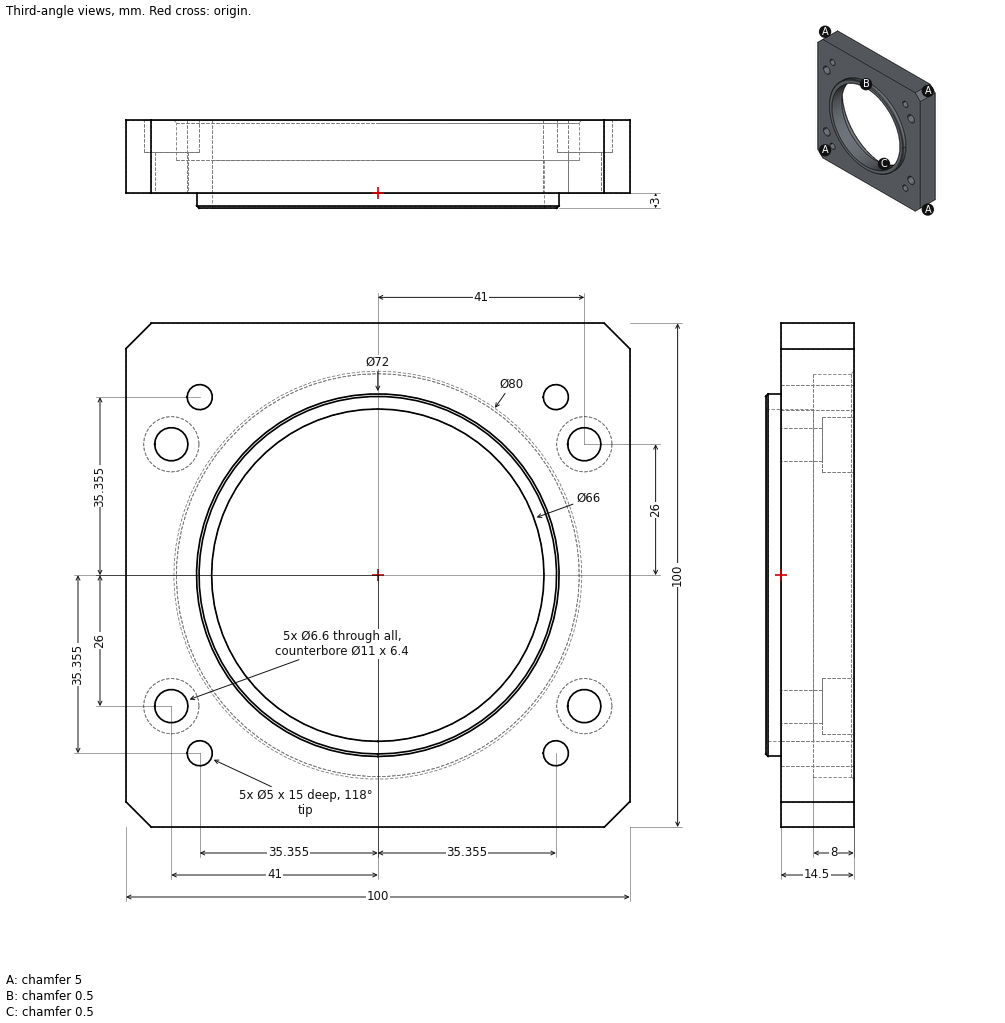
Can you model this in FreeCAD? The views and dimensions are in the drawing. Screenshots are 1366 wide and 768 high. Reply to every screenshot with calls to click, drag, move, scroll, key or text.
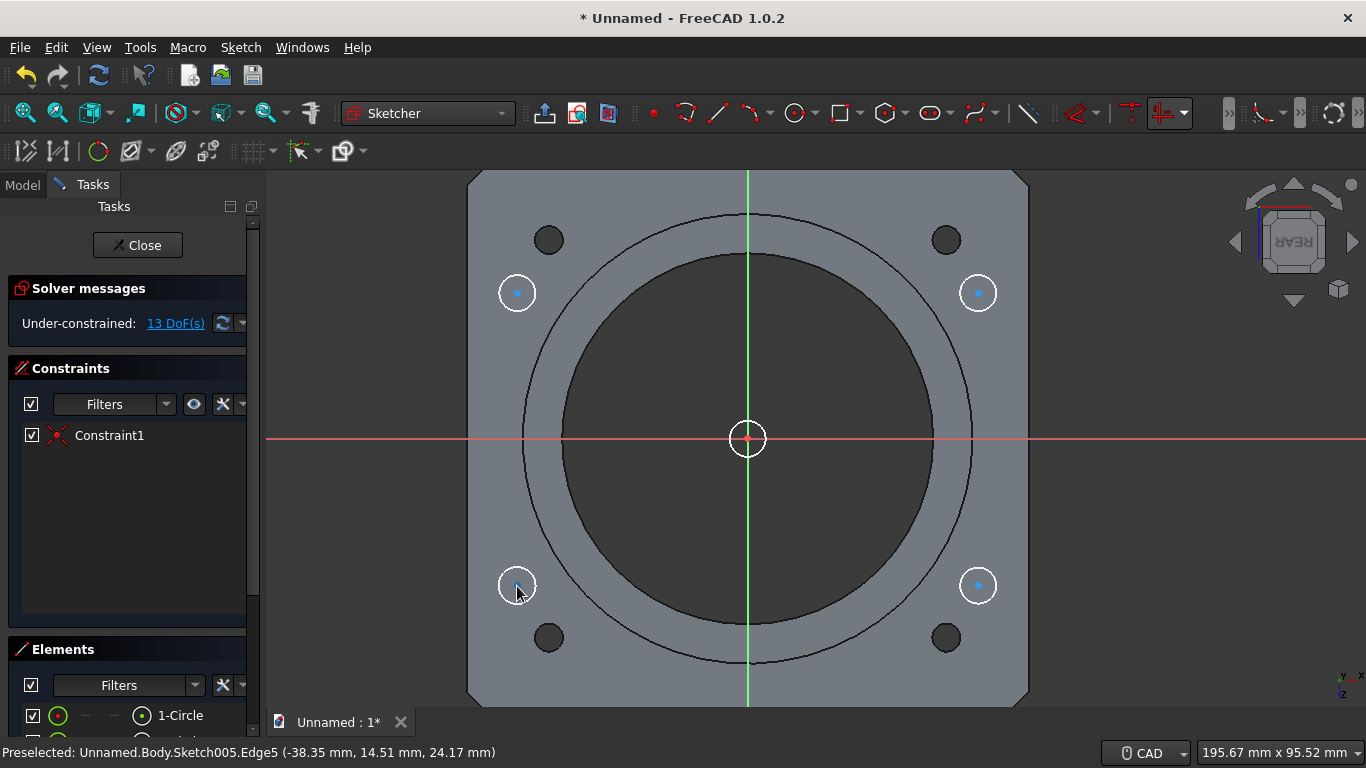
click(530, 280)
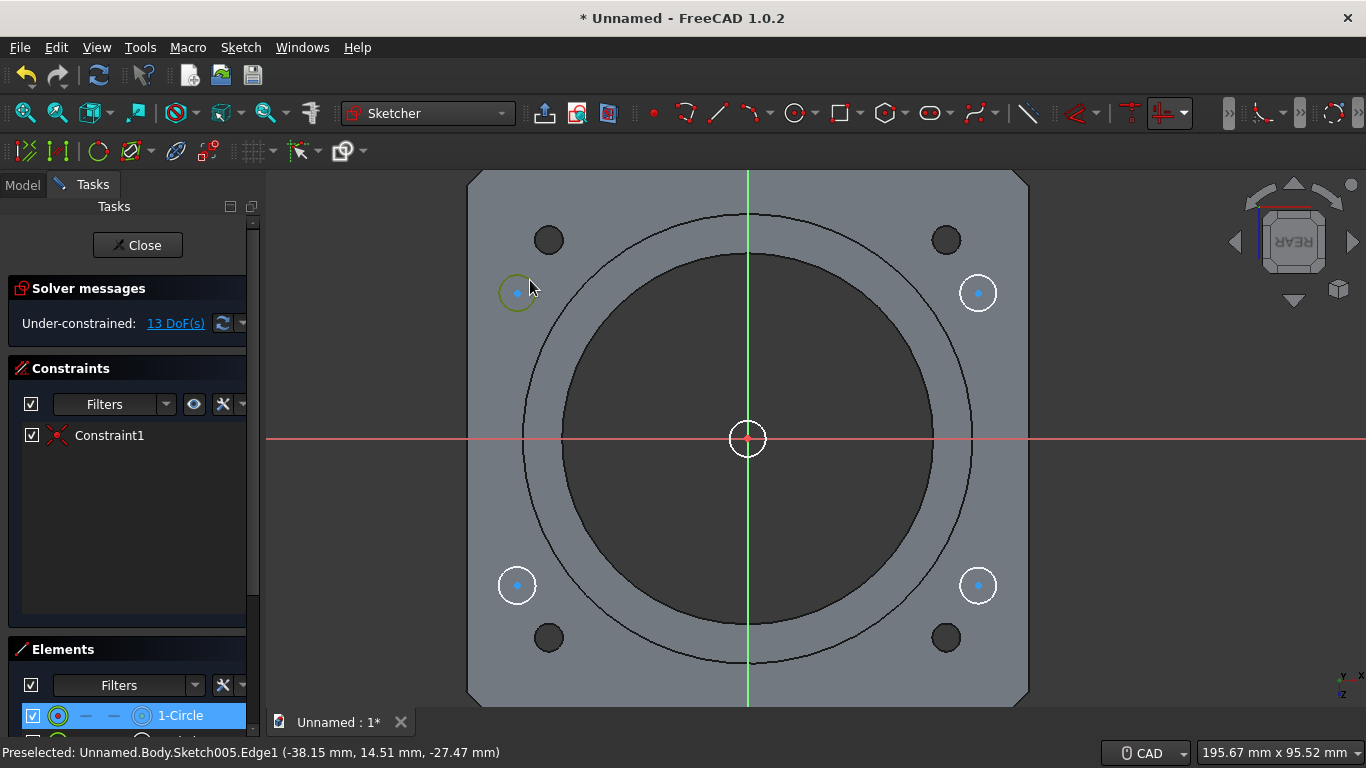
click(760, 426)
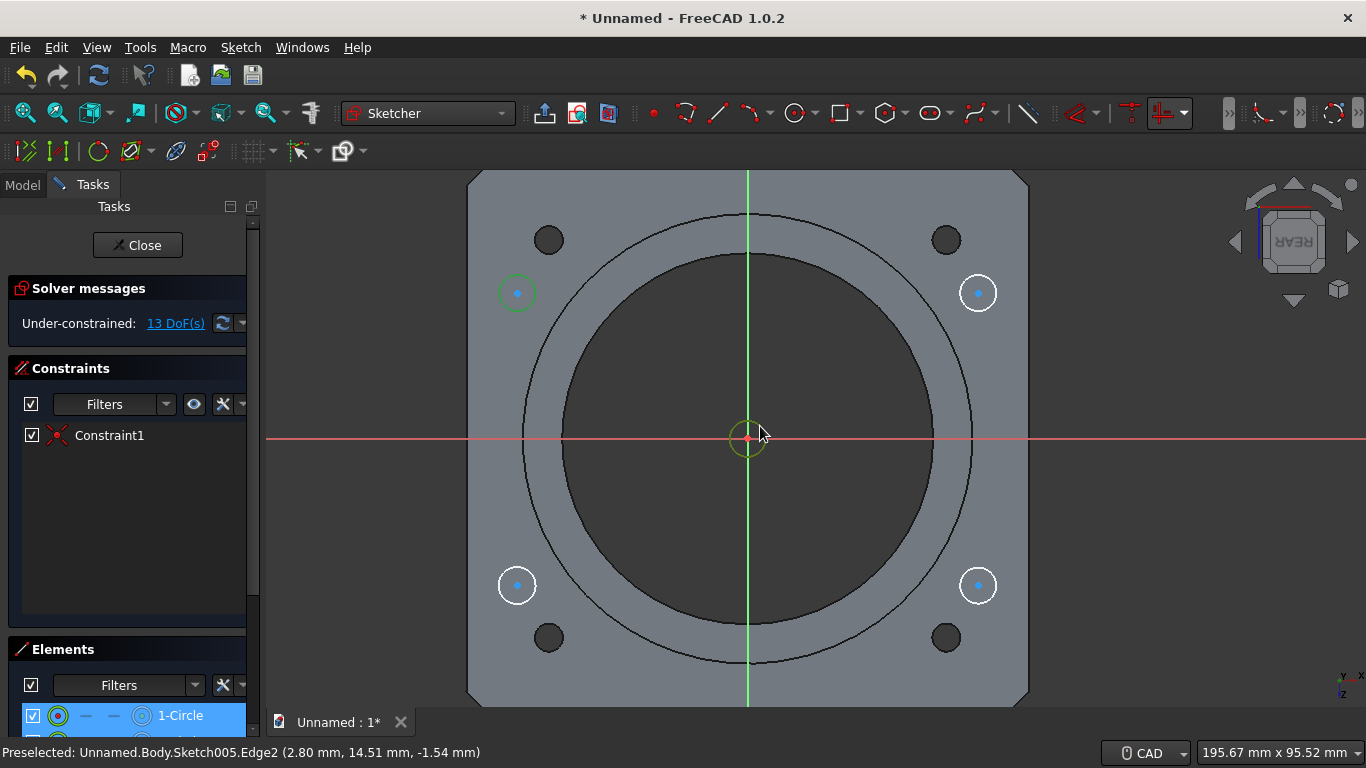
click(991, 573)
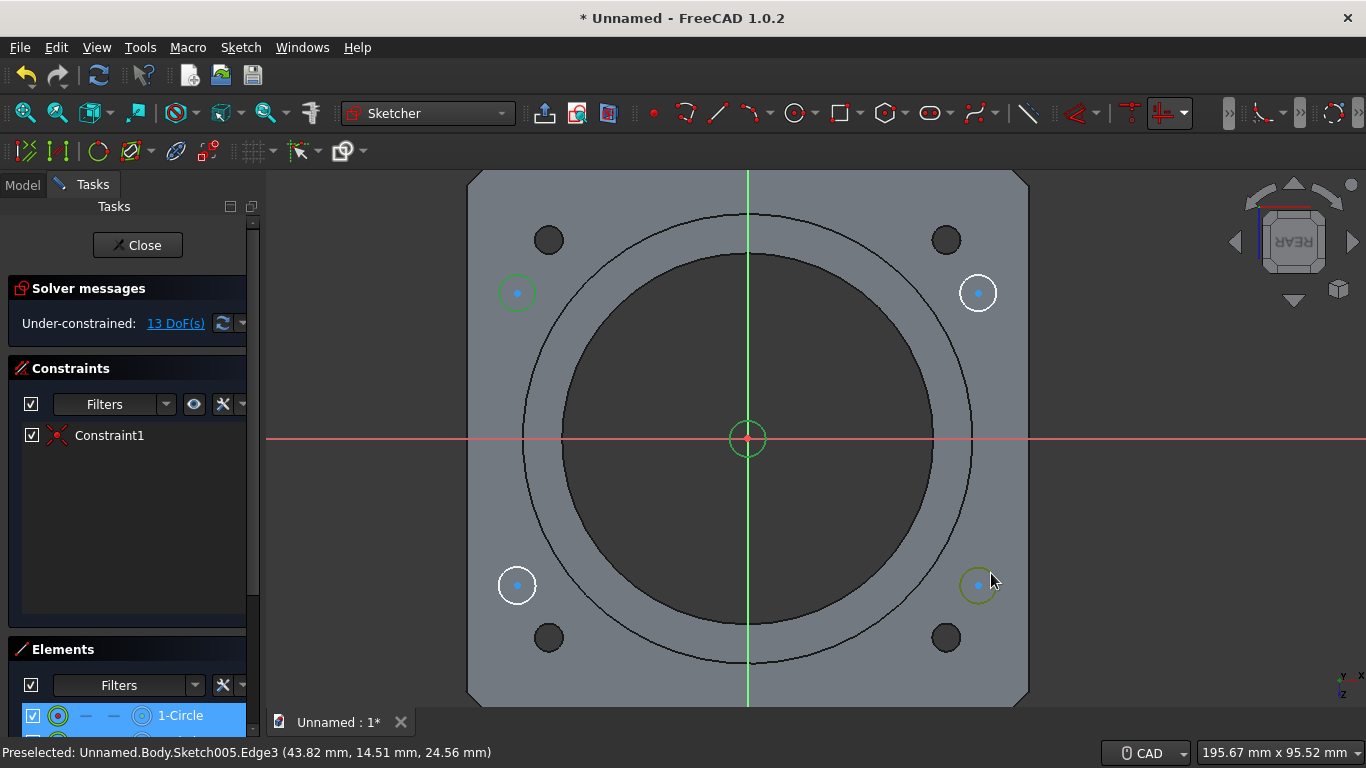
click(991, 280)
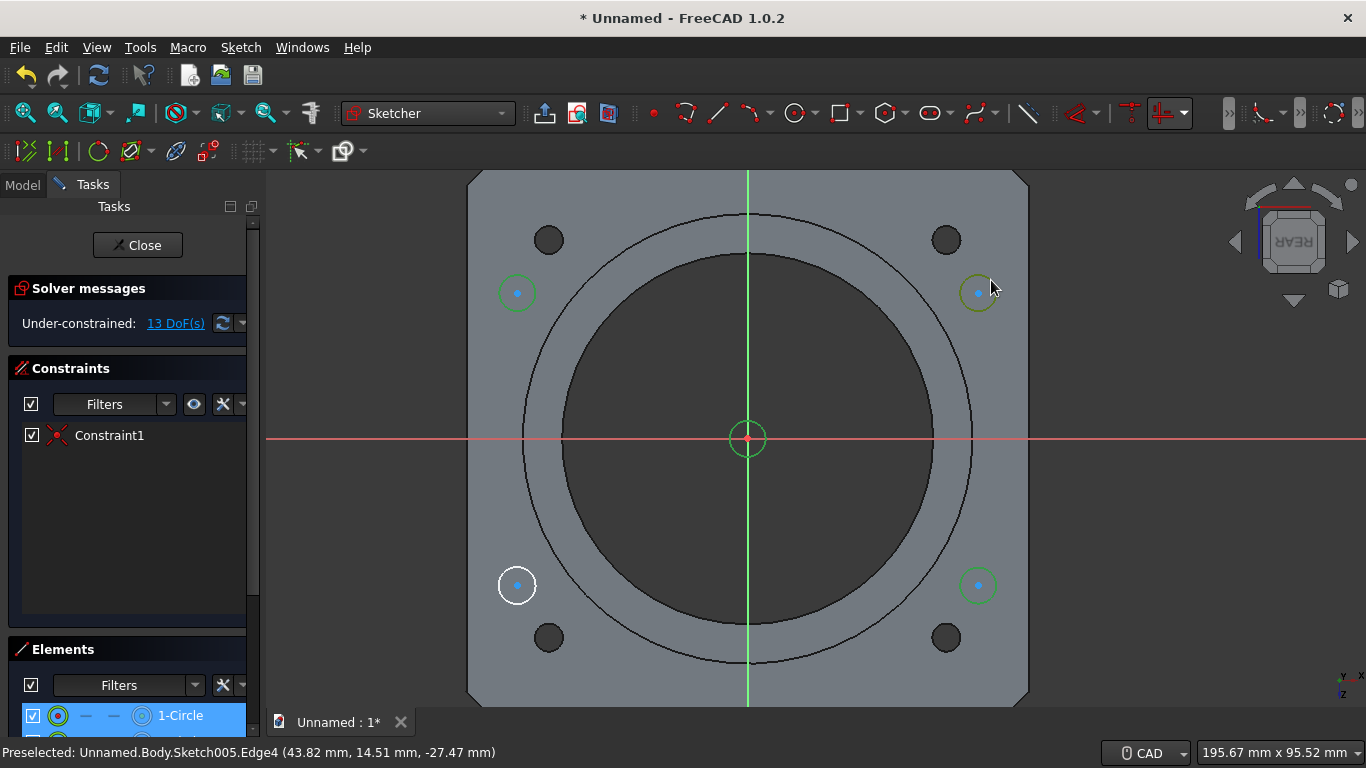
click(530, 572)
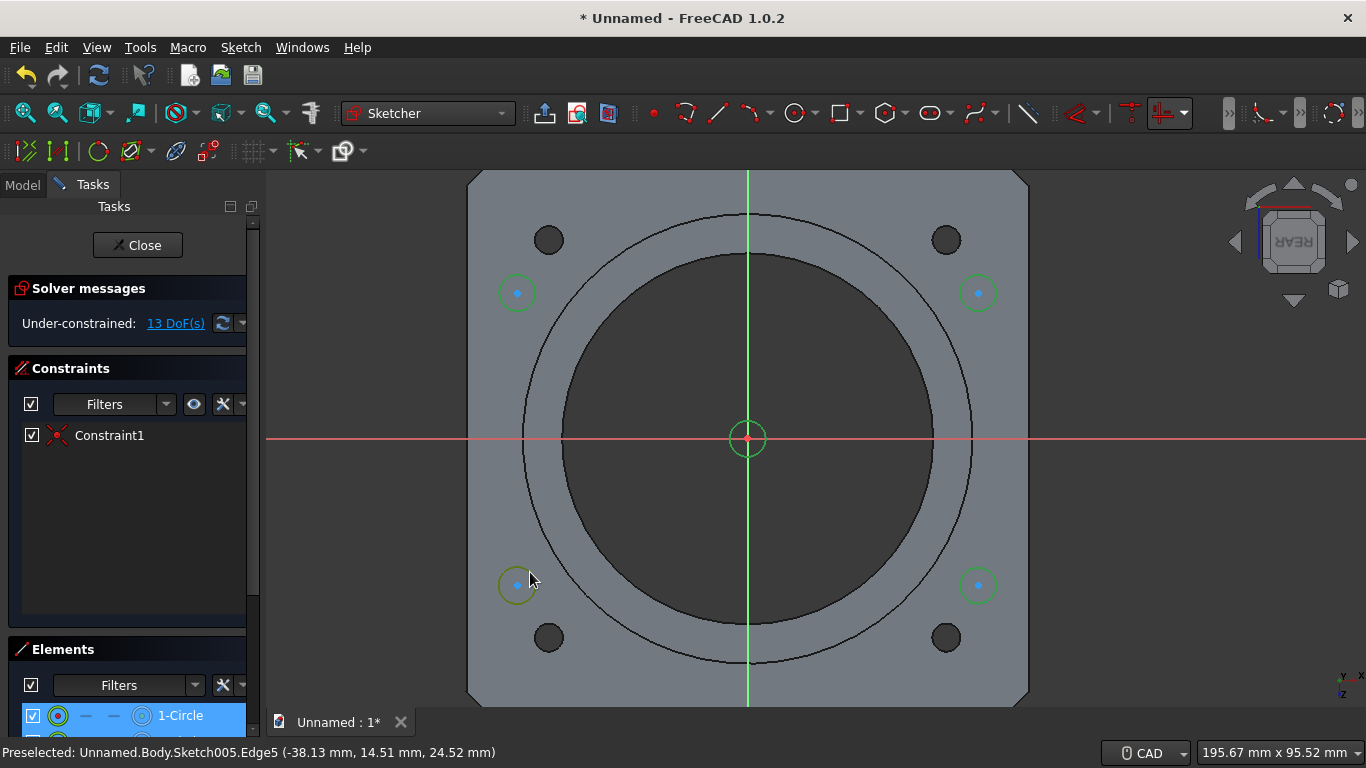
key(e)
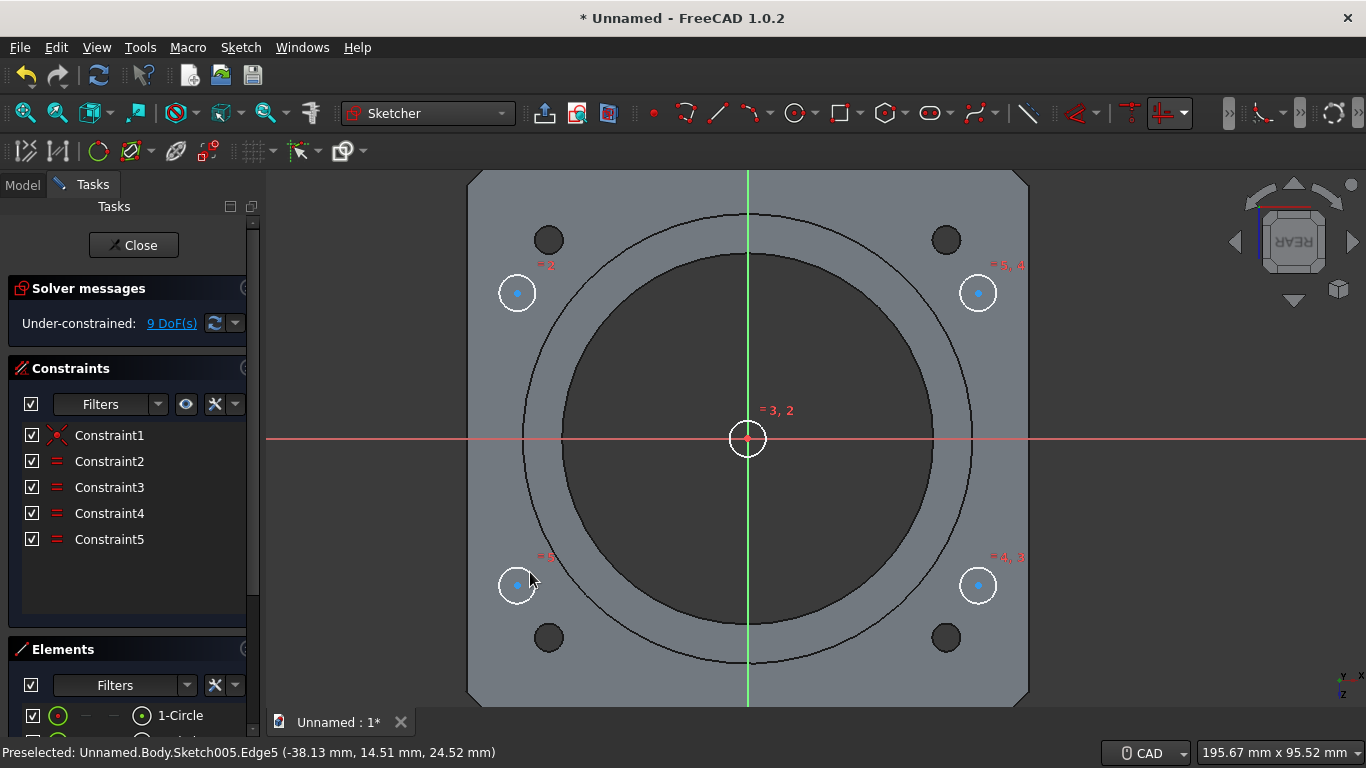
click(978, 586)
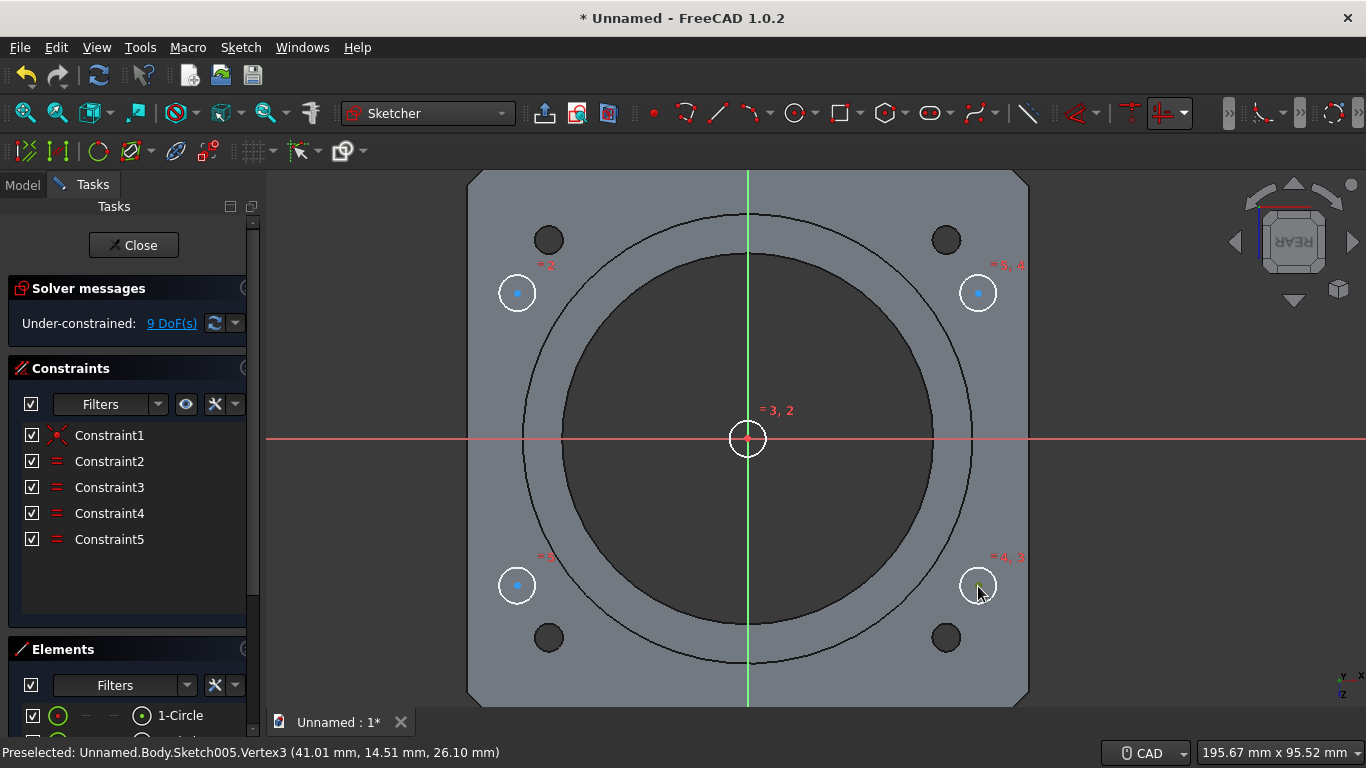
click(978, 293)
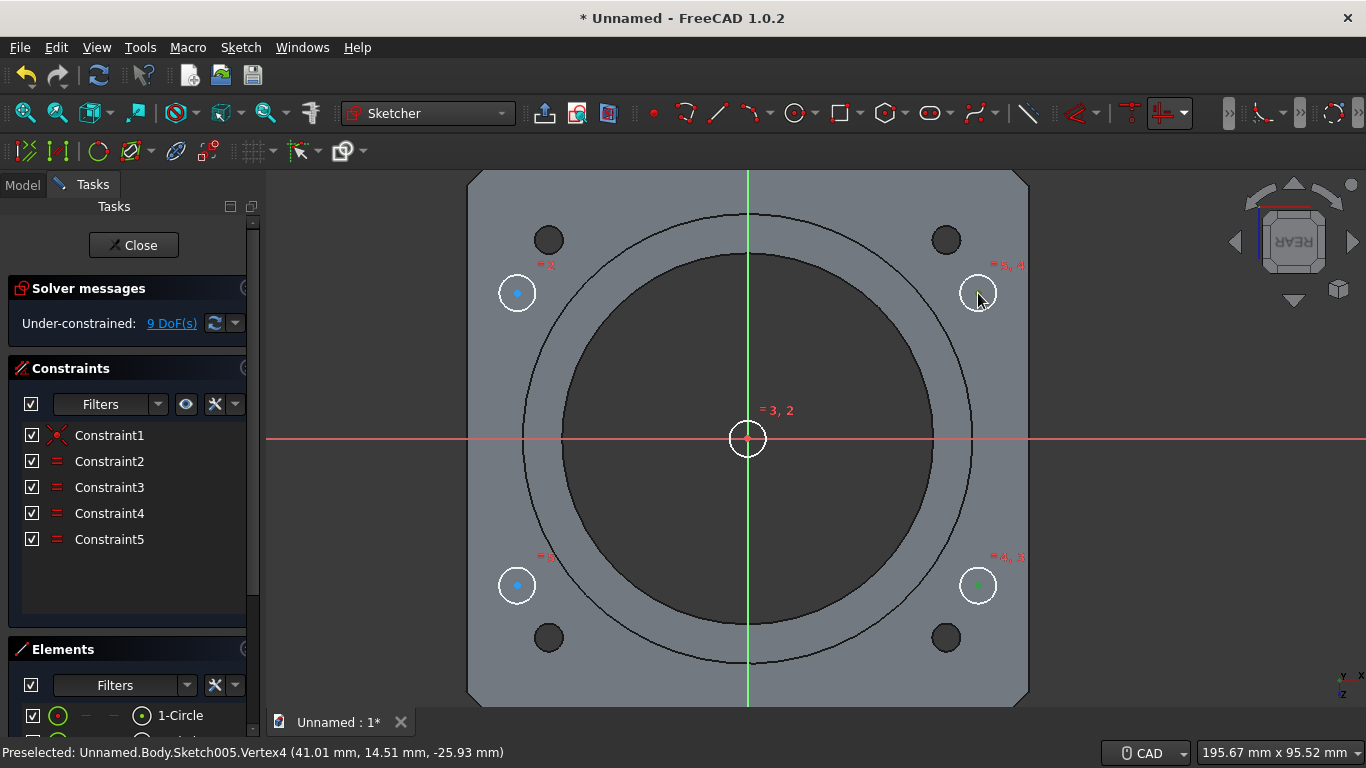
key(v)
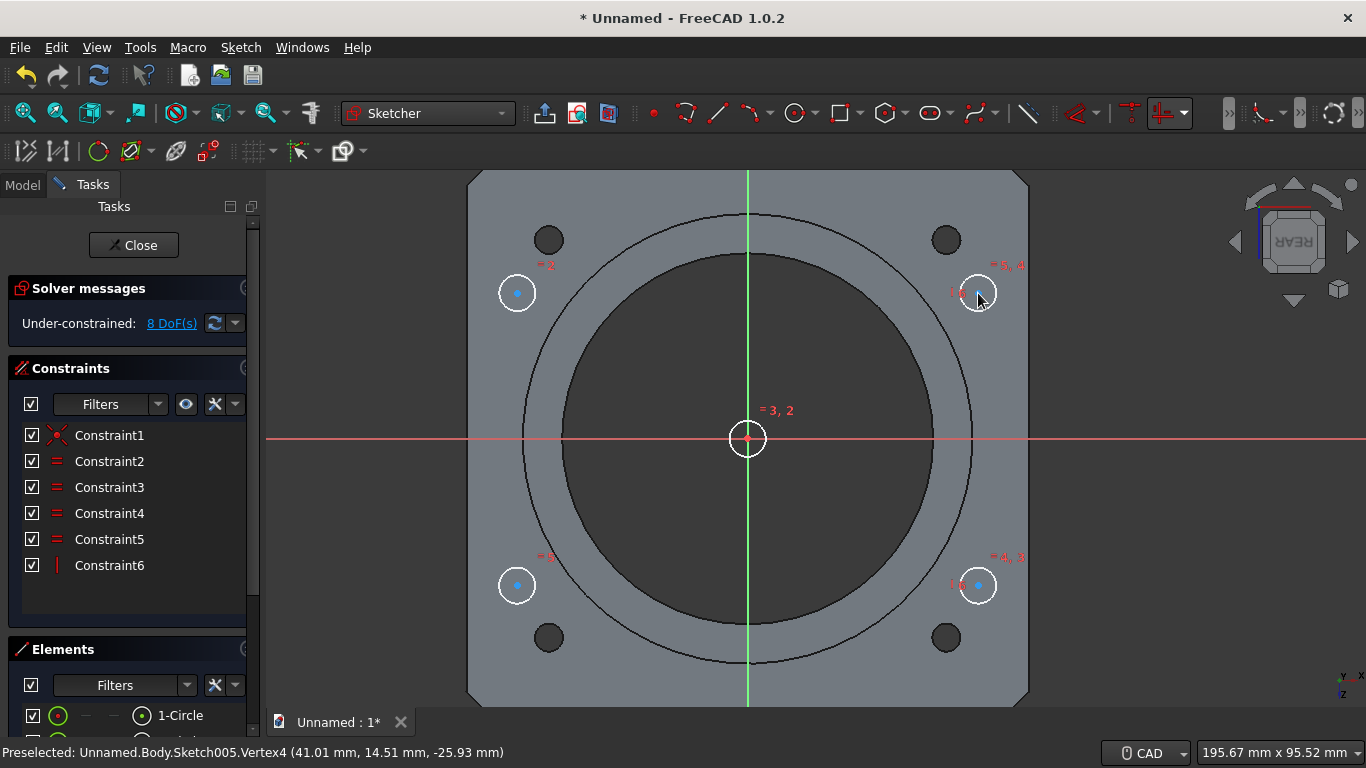
click(517, 293)